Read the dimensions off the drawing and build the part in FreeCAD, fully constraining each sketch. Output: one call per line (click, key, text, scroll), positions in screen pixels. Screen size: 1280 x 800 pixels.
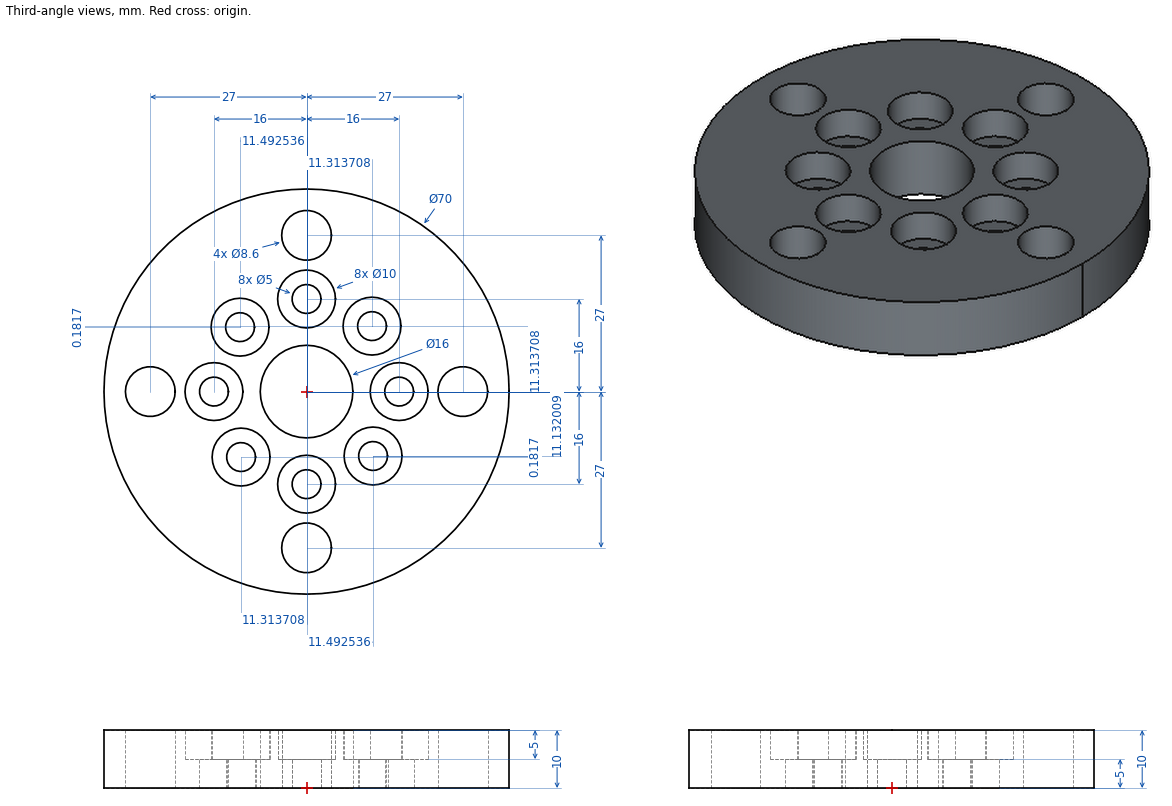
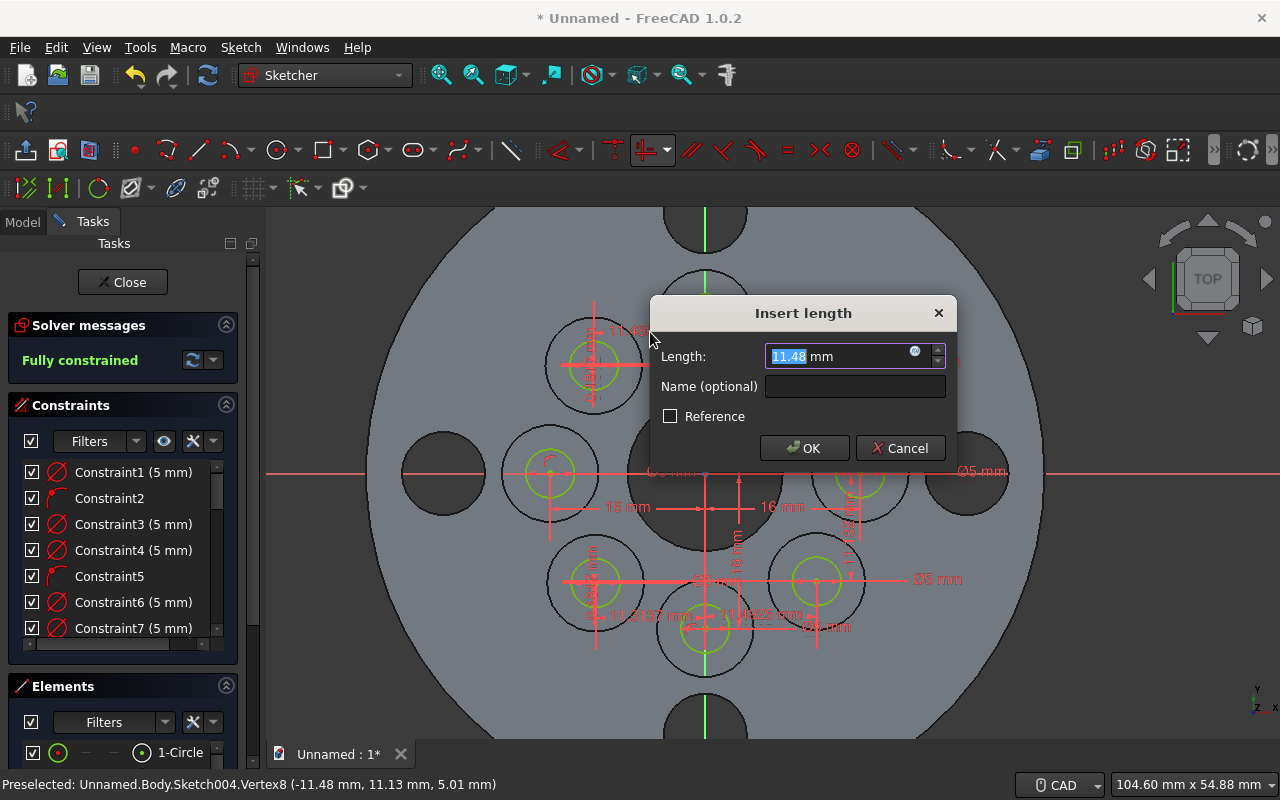
text(11.492536)
key(Return)
key(Escape)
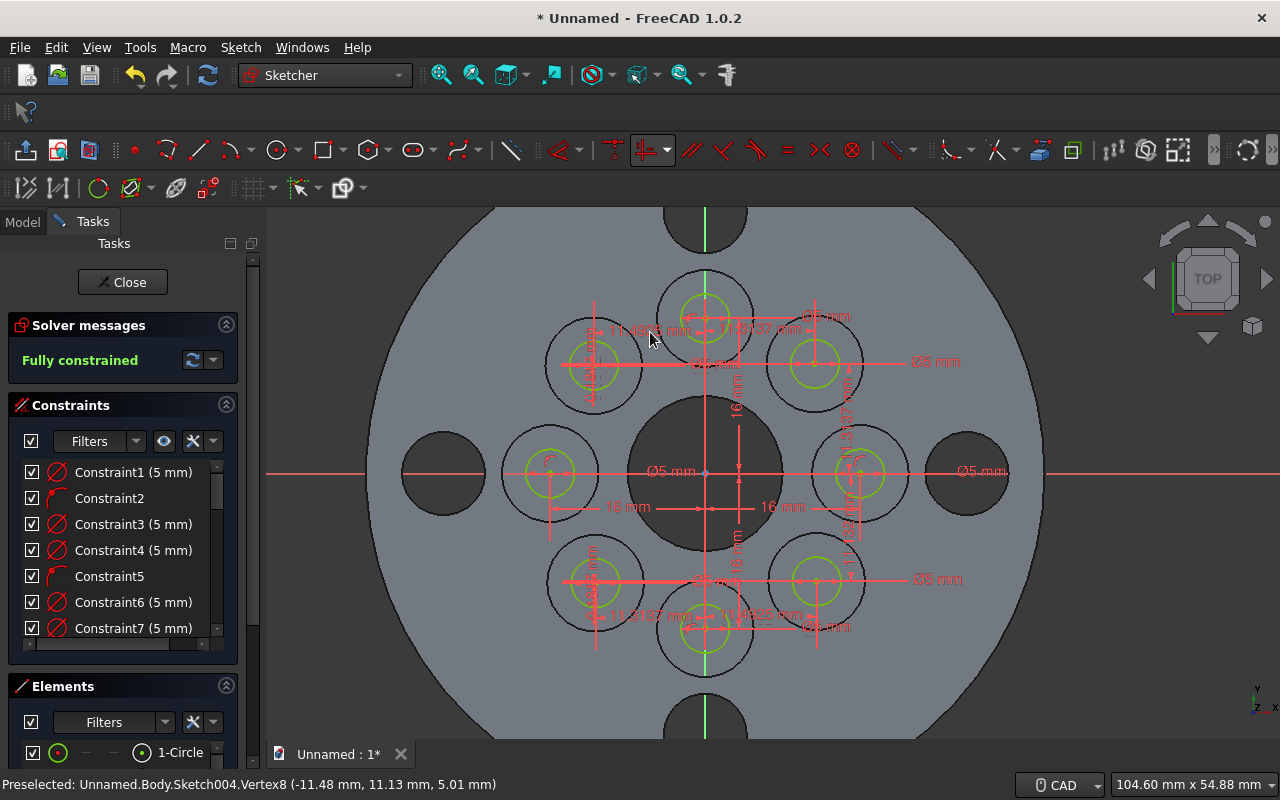
click(123, 282)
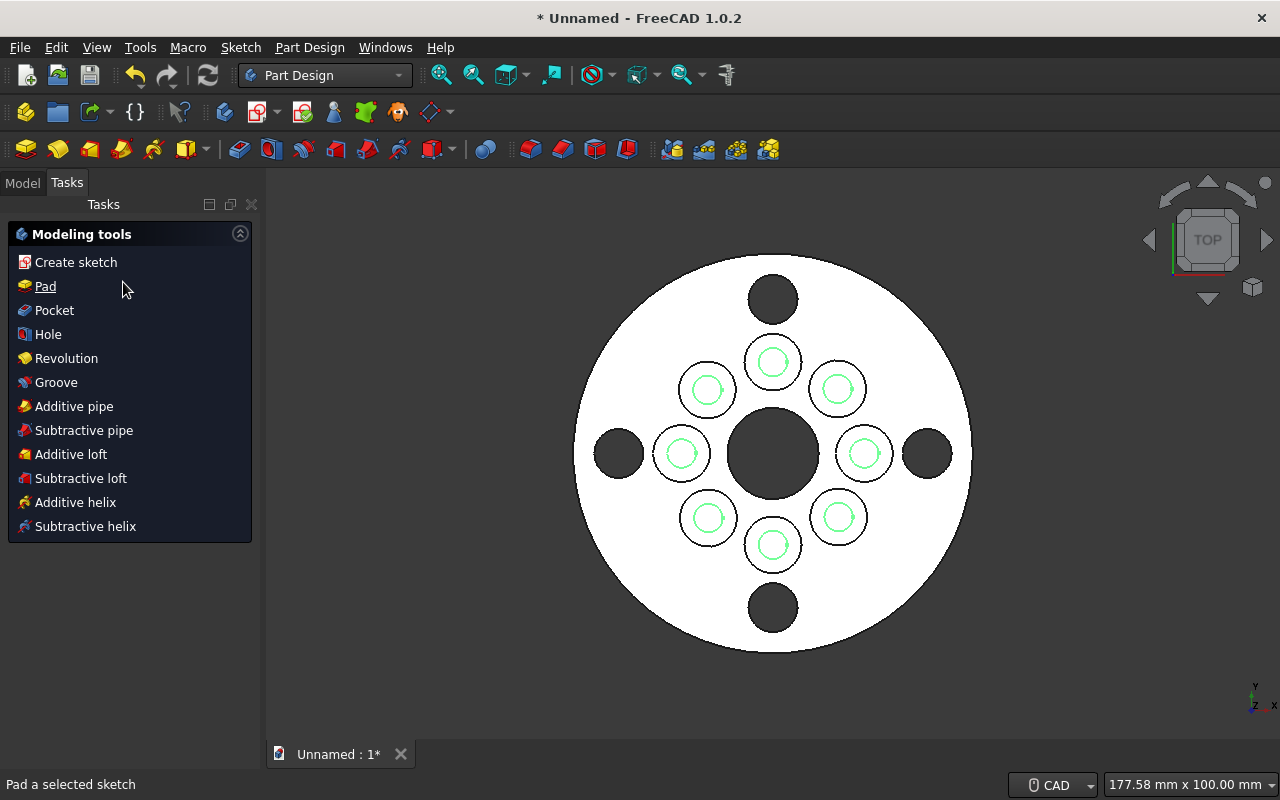
click(240, 150)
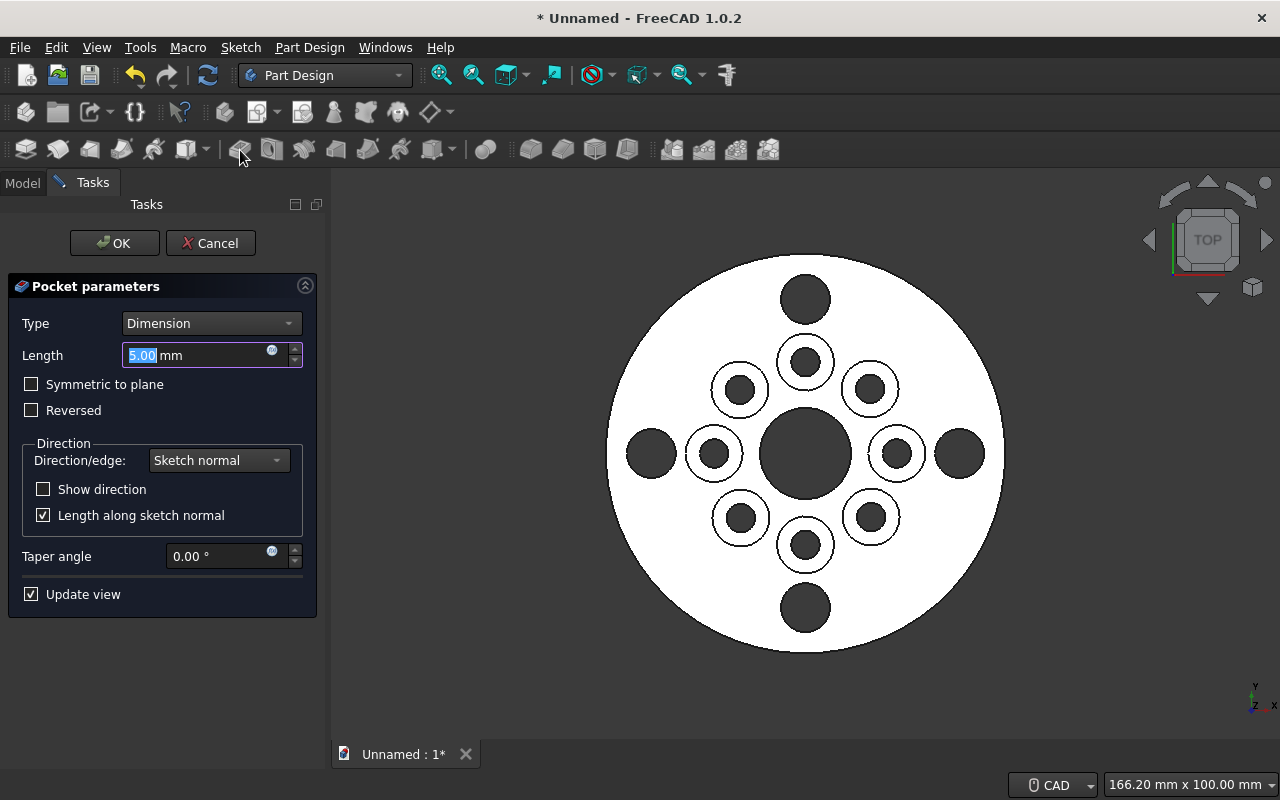
text(5)
key(Tab)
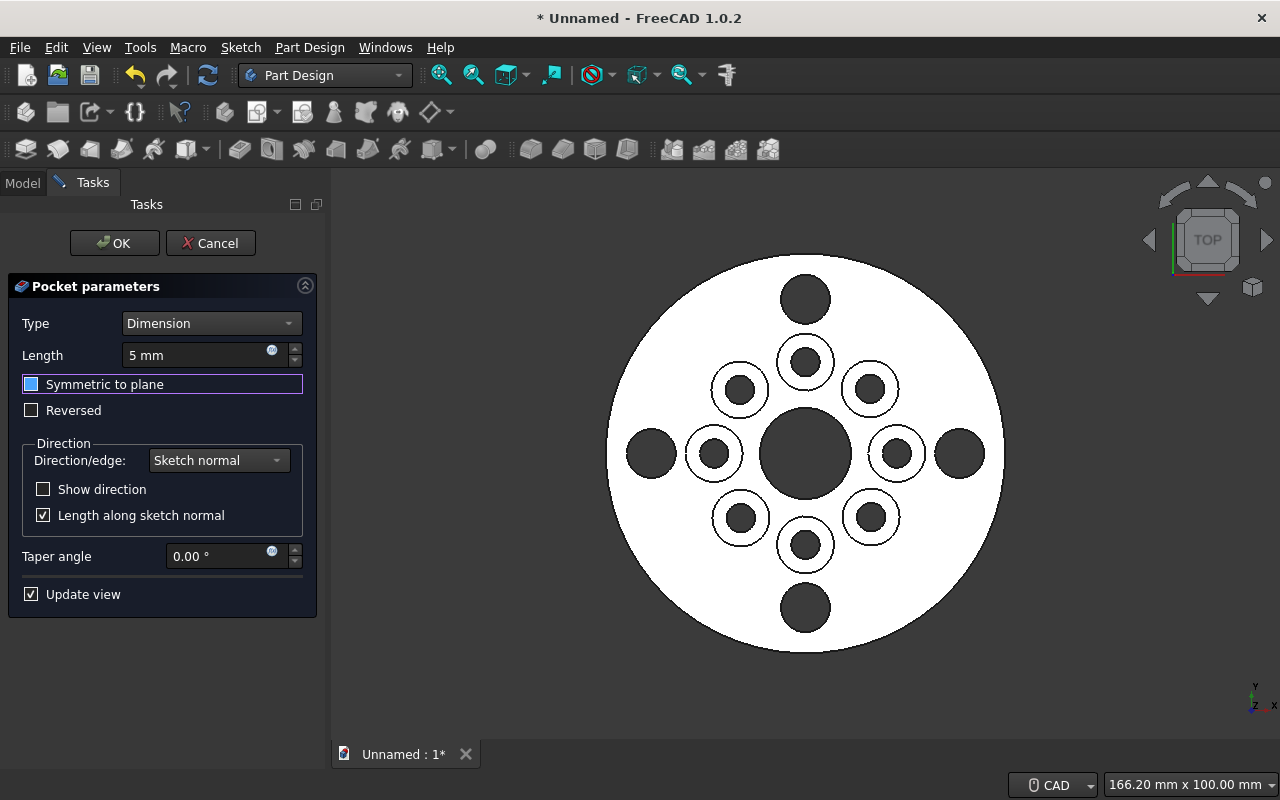
click(115, 243)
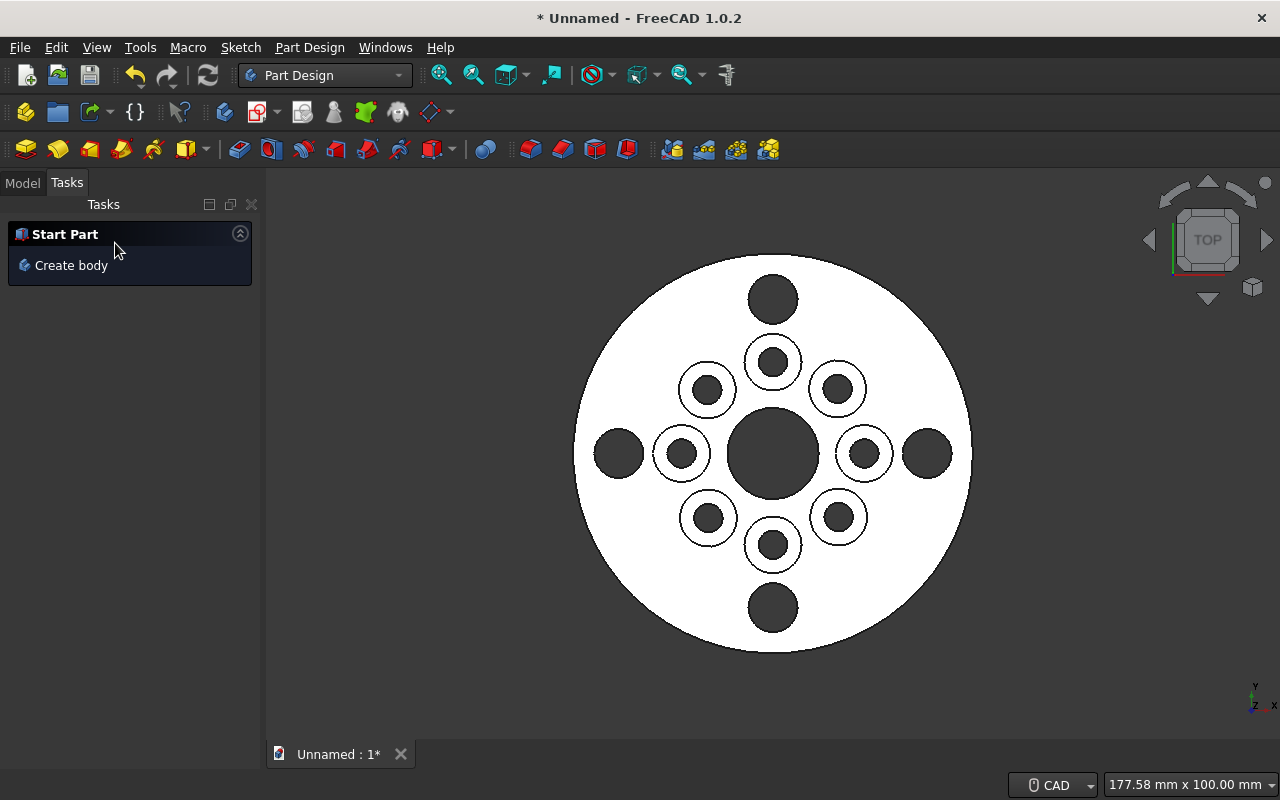
key(0)